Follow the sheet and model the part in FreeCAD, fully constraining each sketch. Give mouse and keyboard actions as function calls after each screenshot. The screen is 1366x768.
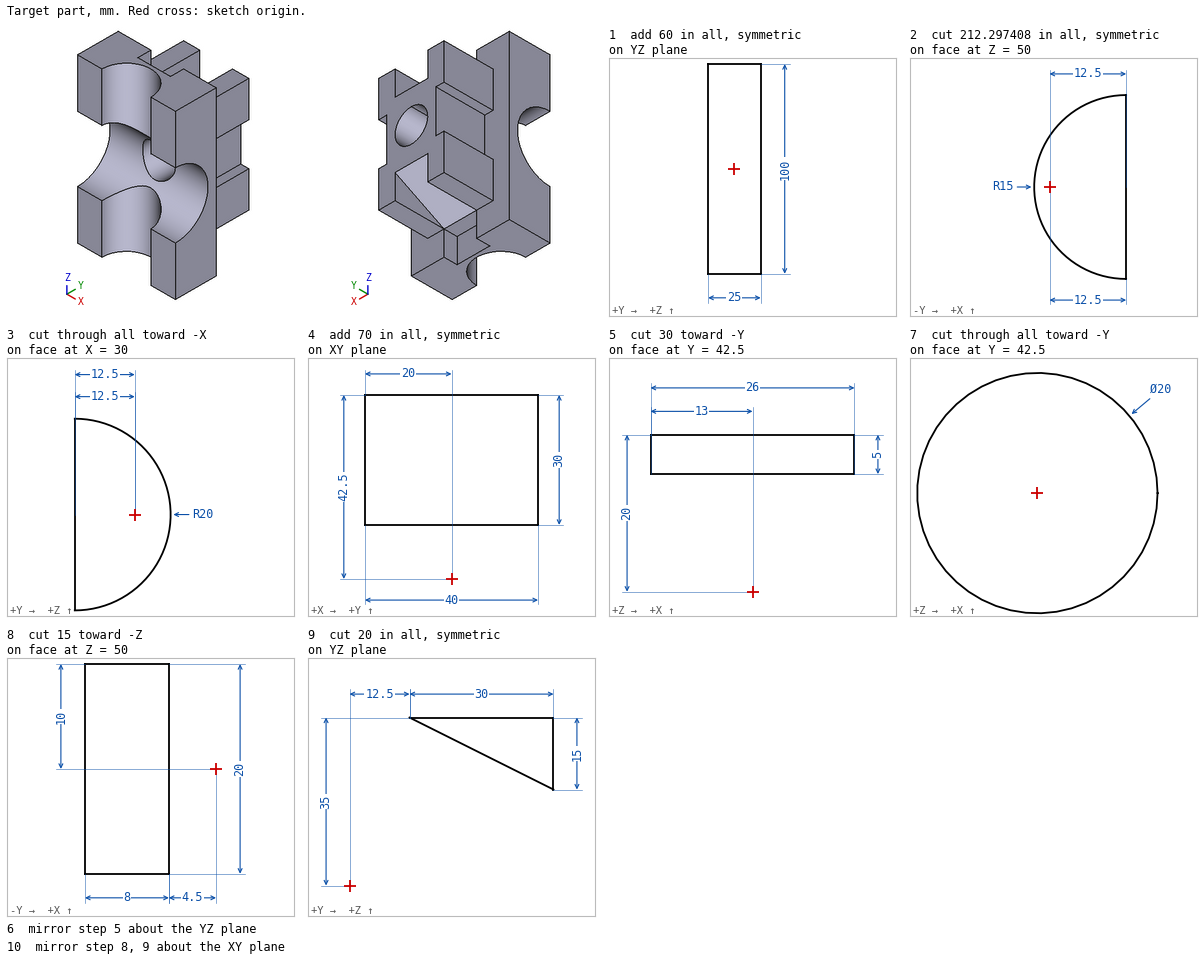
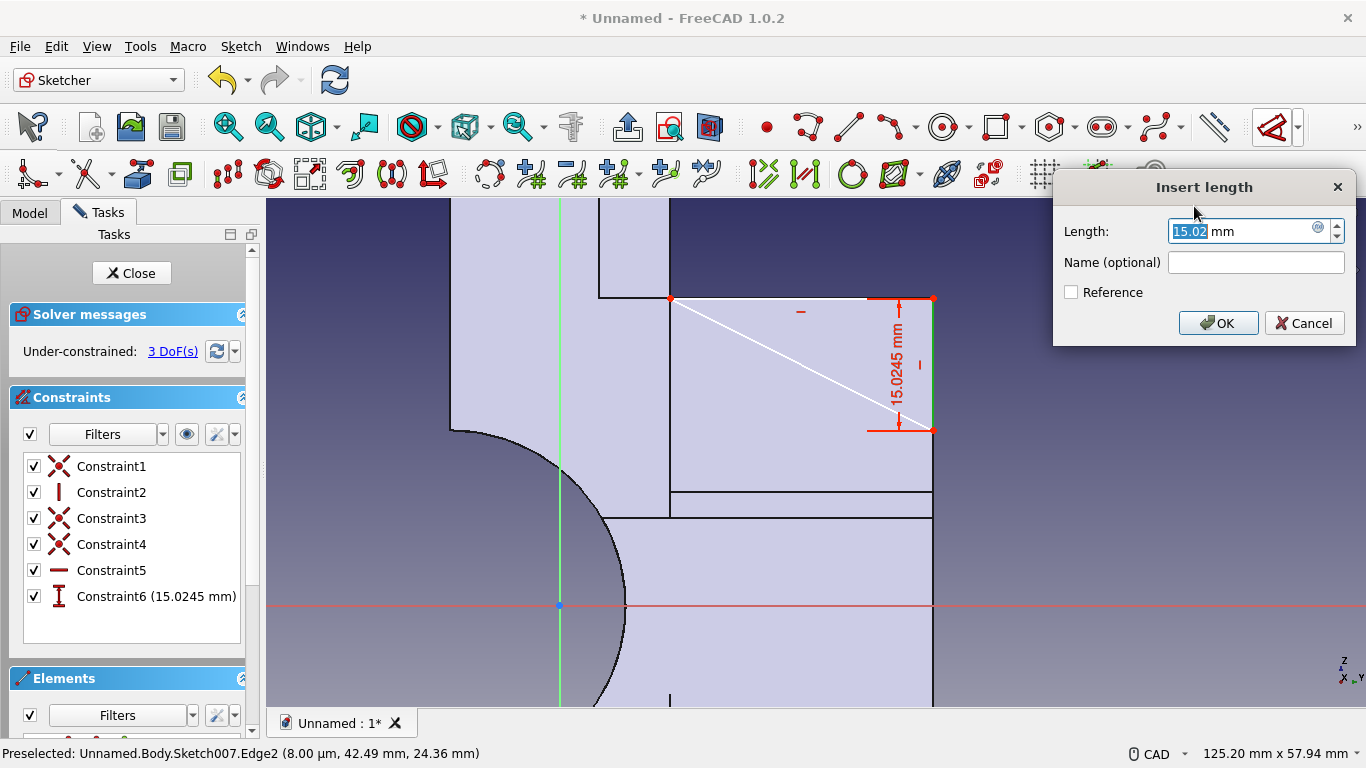
text(15)
key(Return)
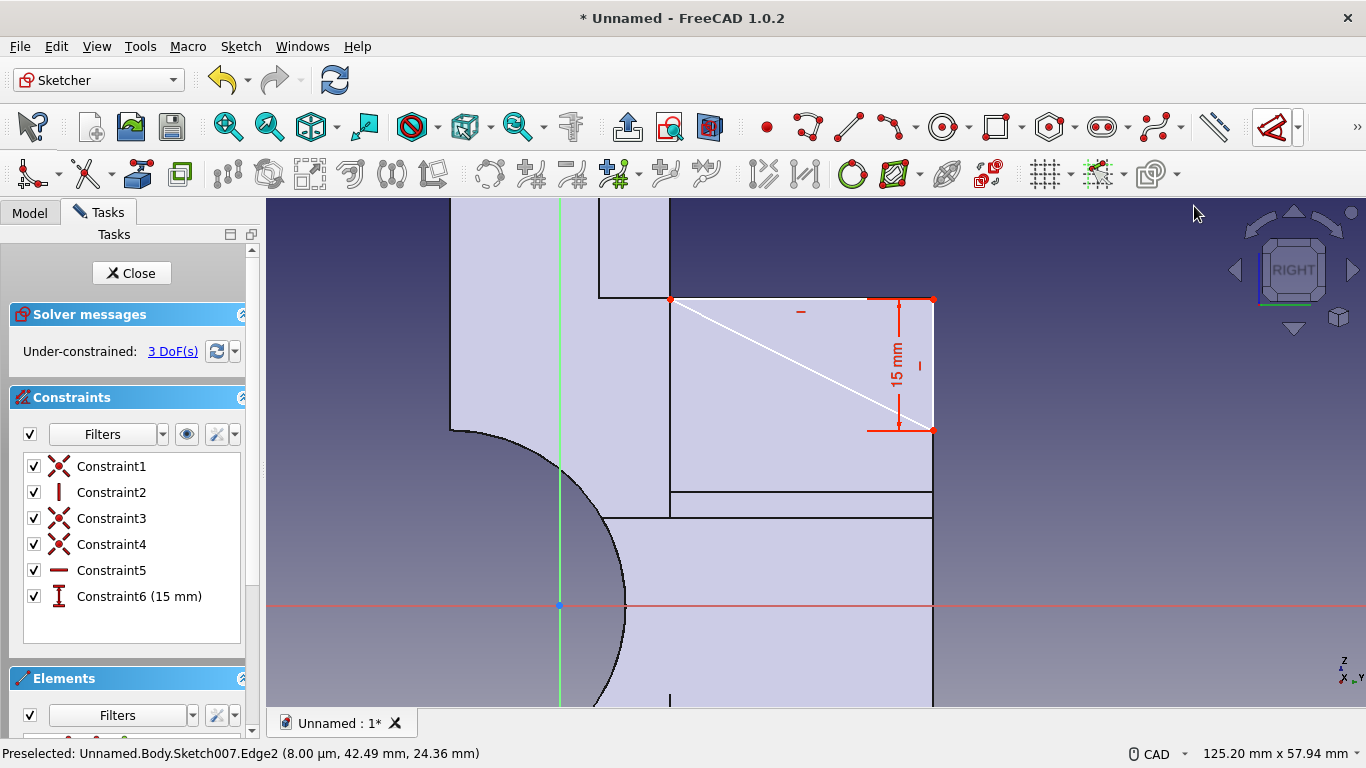
click(854, 299)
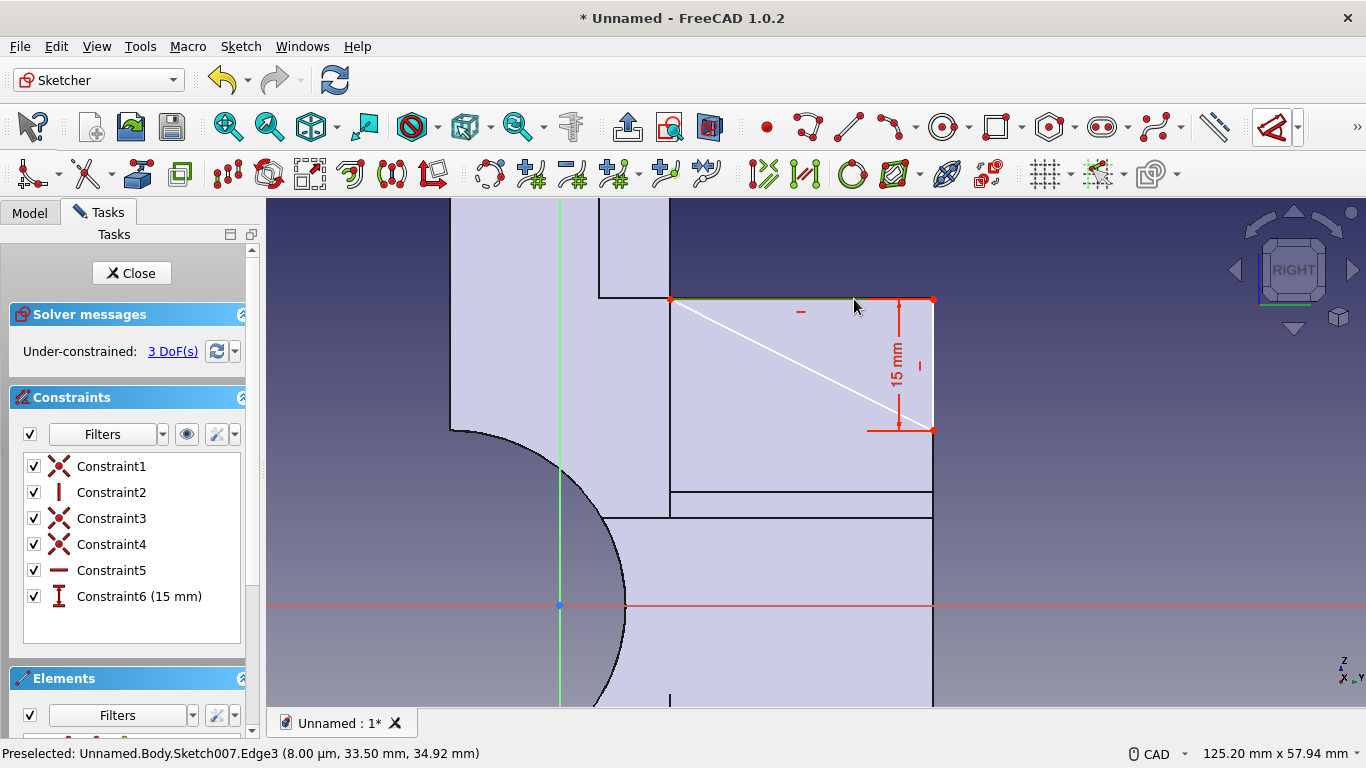
key(l)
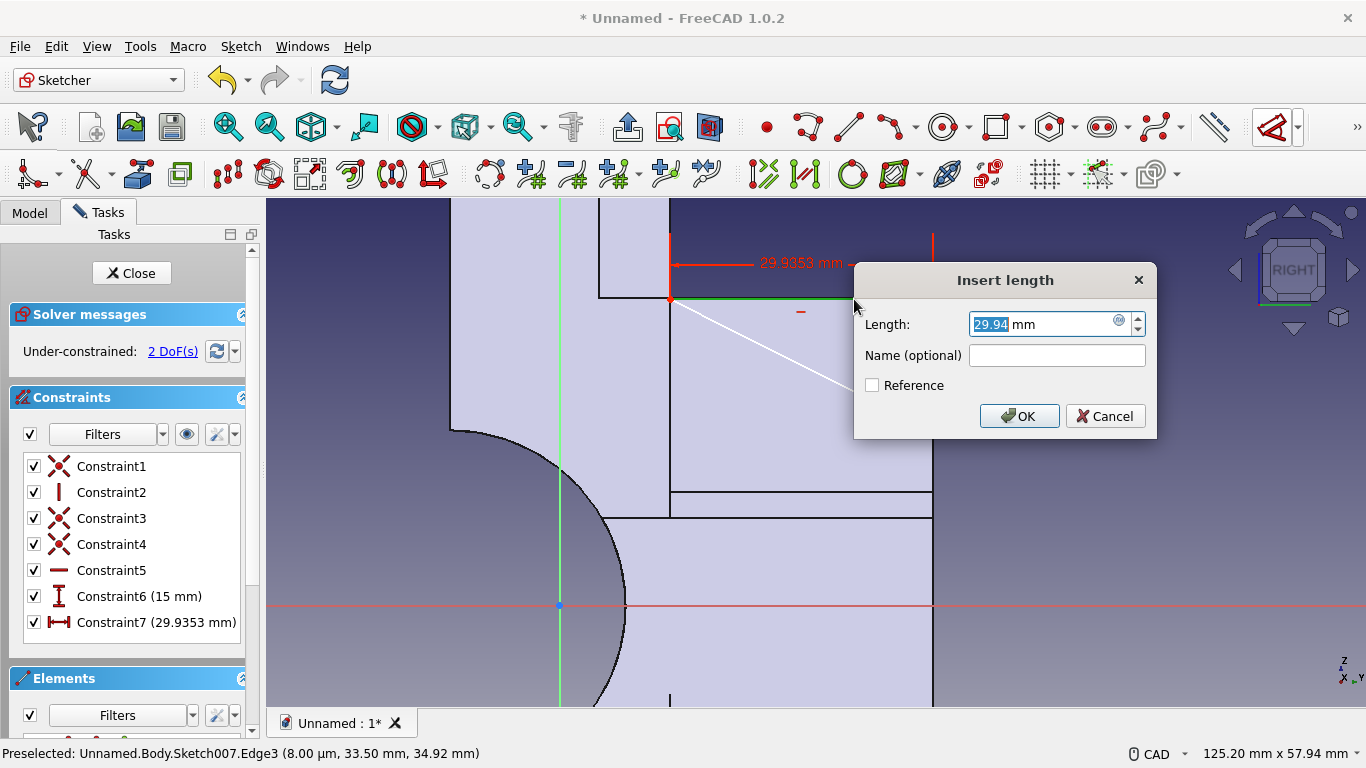
text(30)
key(Return)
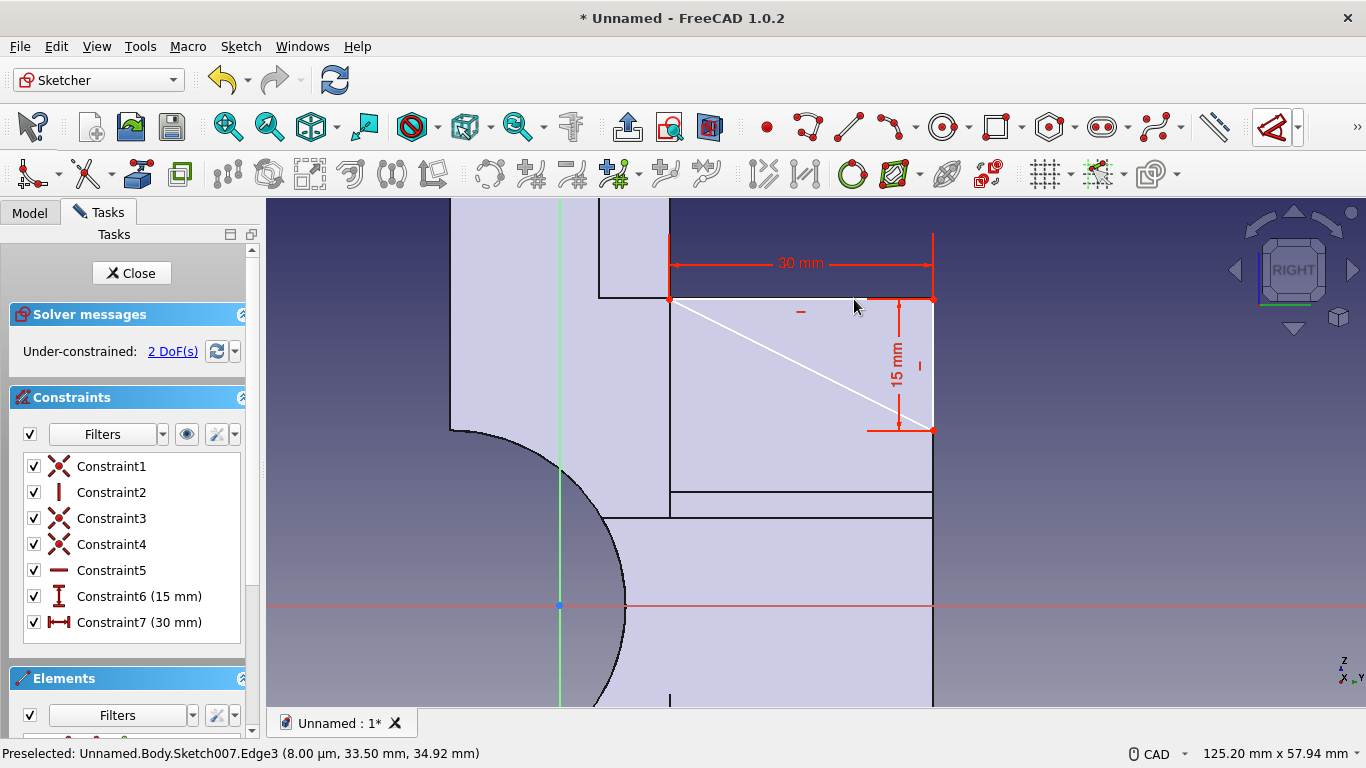
click(669, 299)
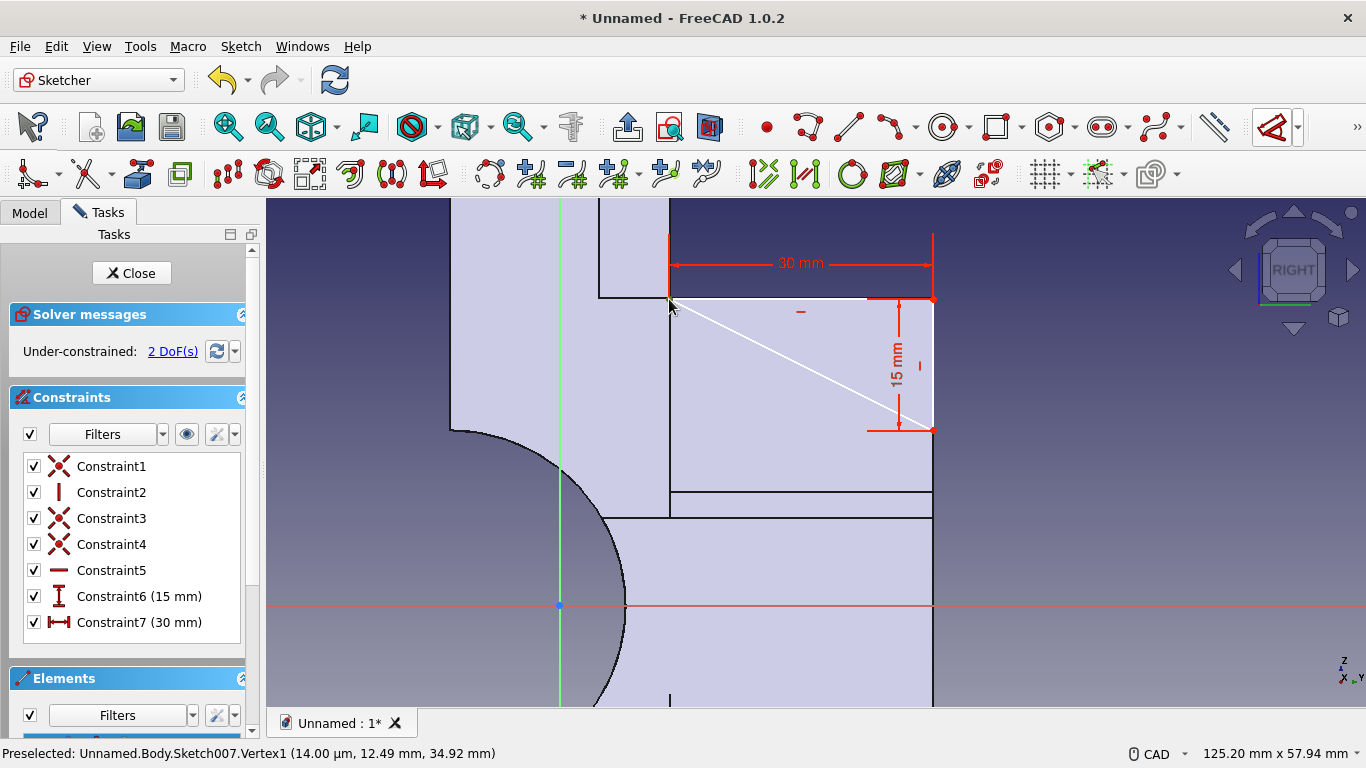
click(1298, 128)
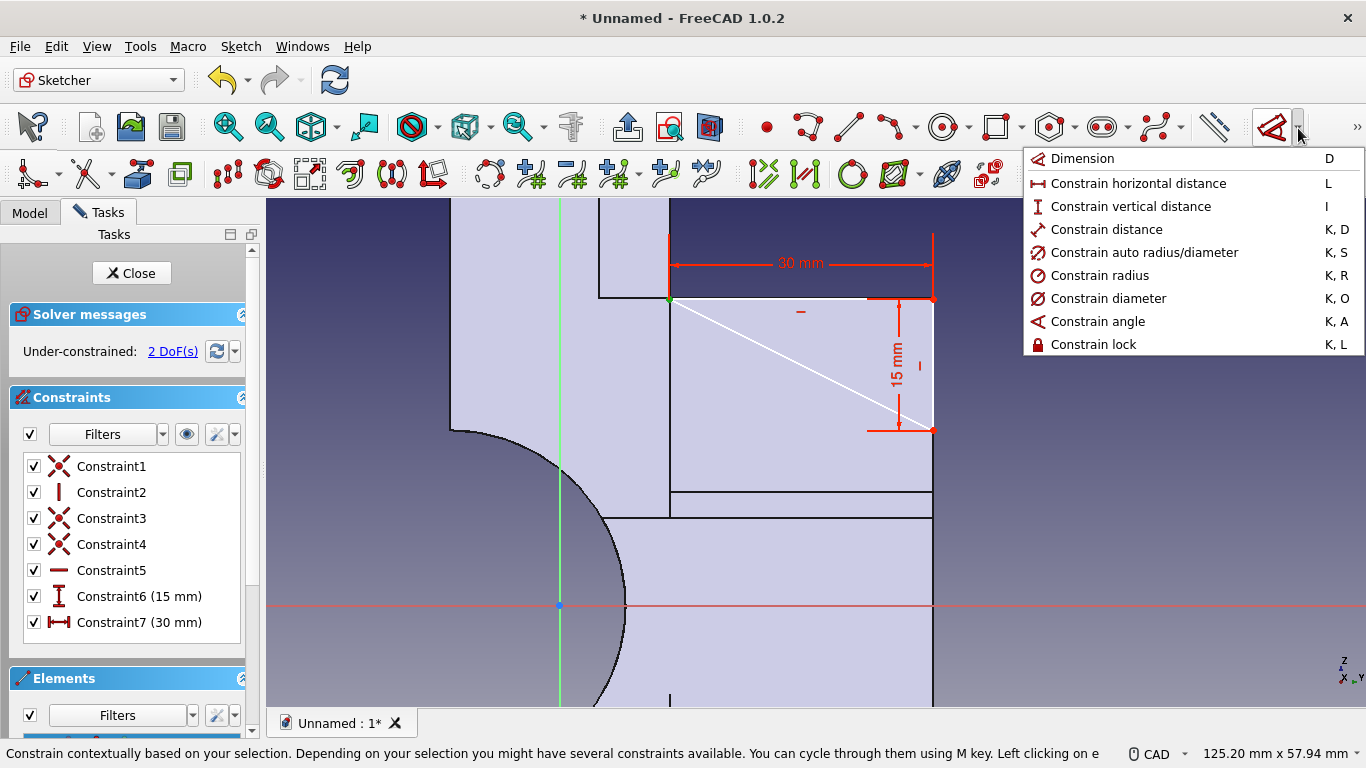
click(1194, 206)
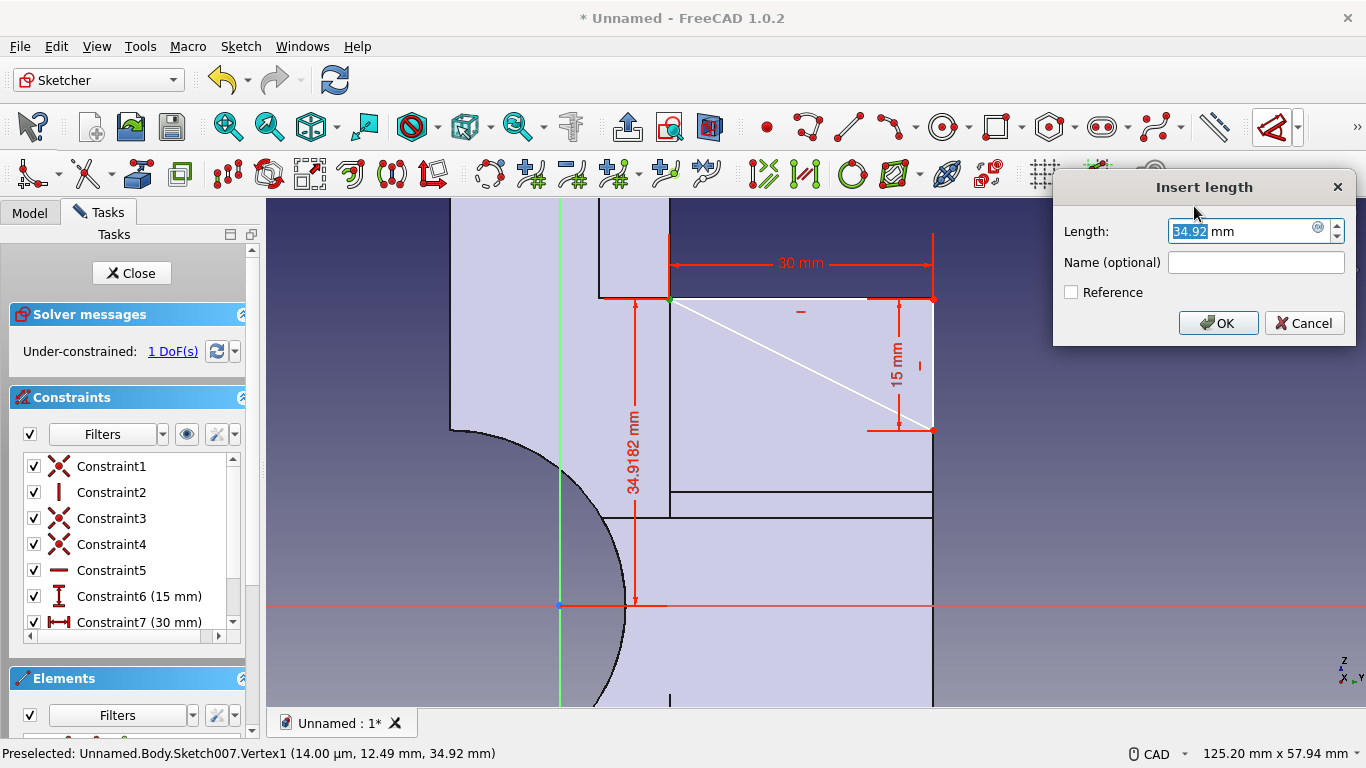
text(35)
key(Return)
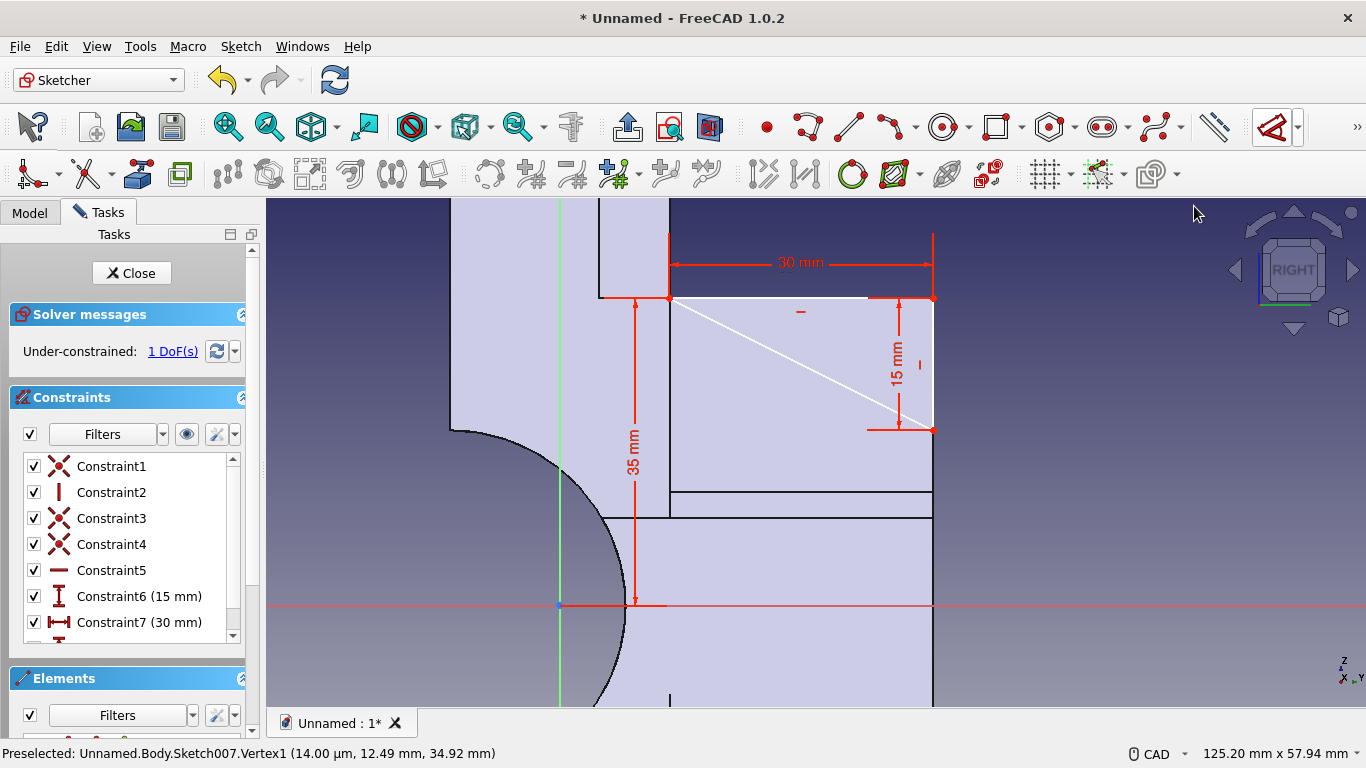
click(669, 298)